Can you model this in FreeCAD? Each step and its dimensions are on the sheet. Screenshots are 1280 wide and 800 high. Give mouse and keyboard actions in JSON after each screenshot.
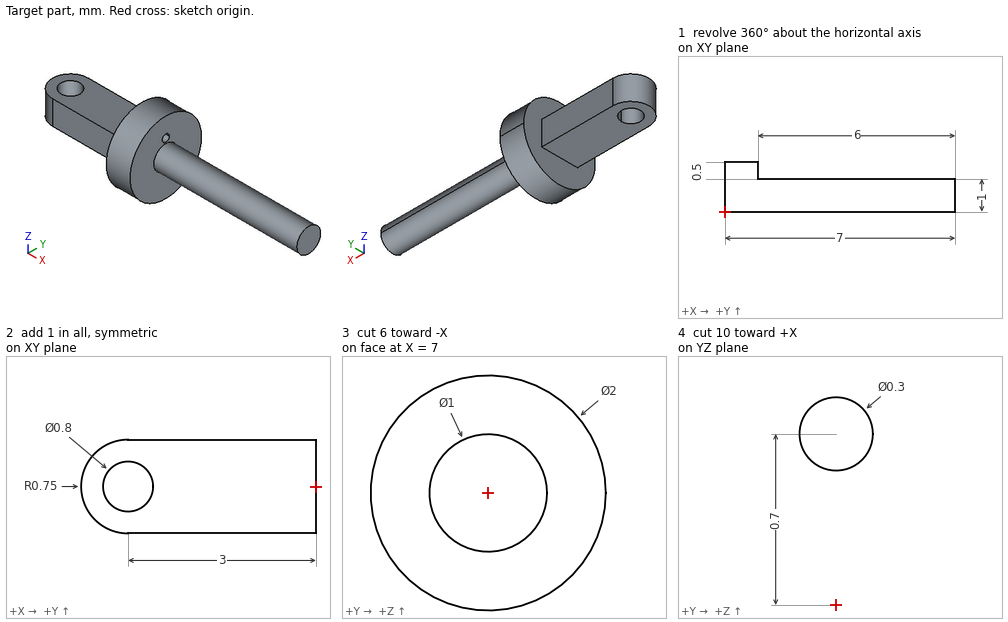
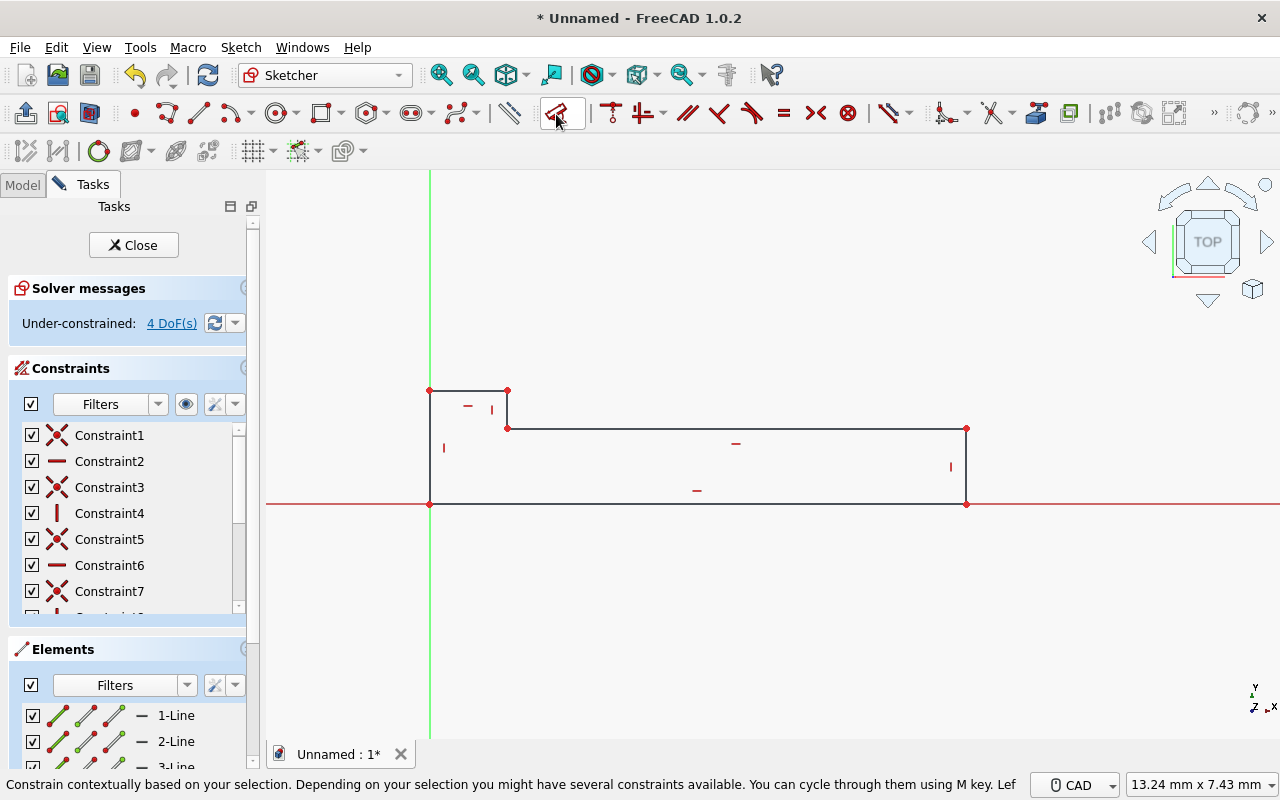
{"action": "left_click", "coordinate": [591, 504]}
{"action": "left_click", "coordinate": [698, 538]}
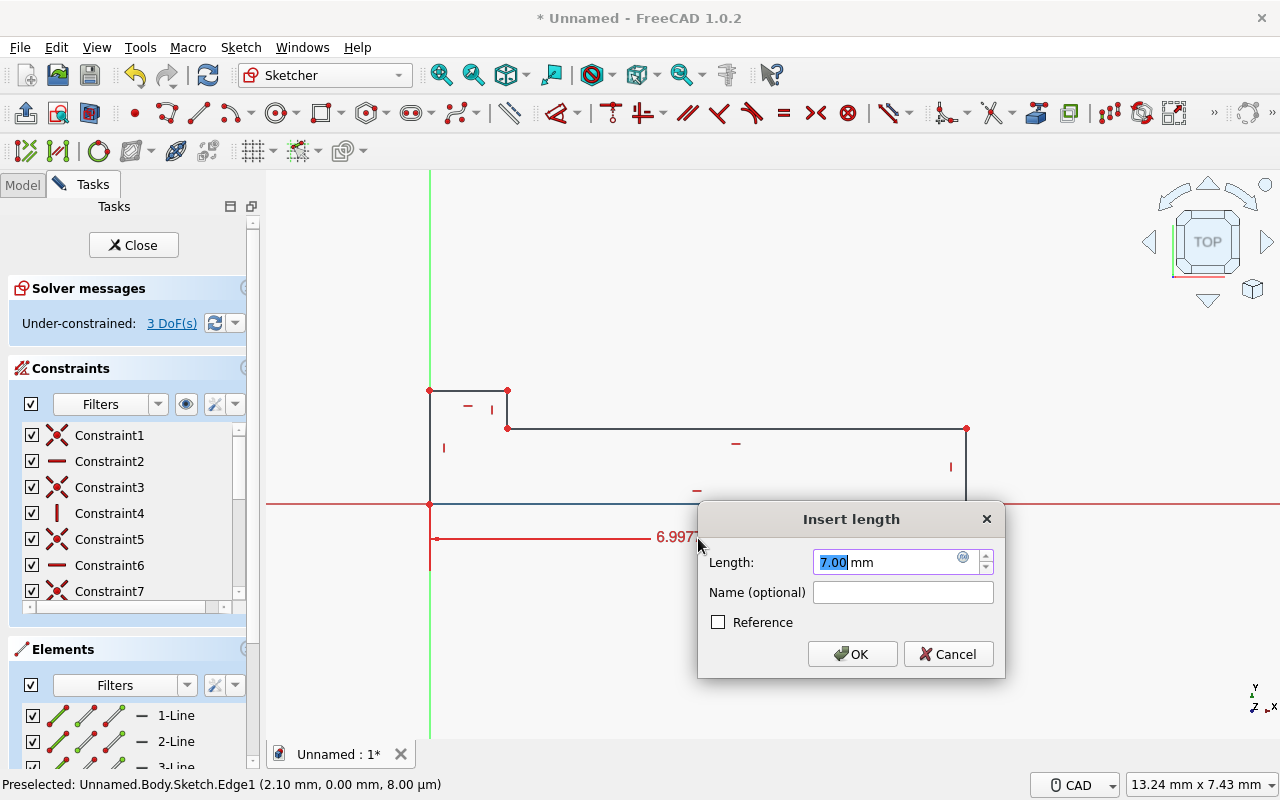
{"action": "type", "text": "7"}
{"action": "key", "text": "Return"}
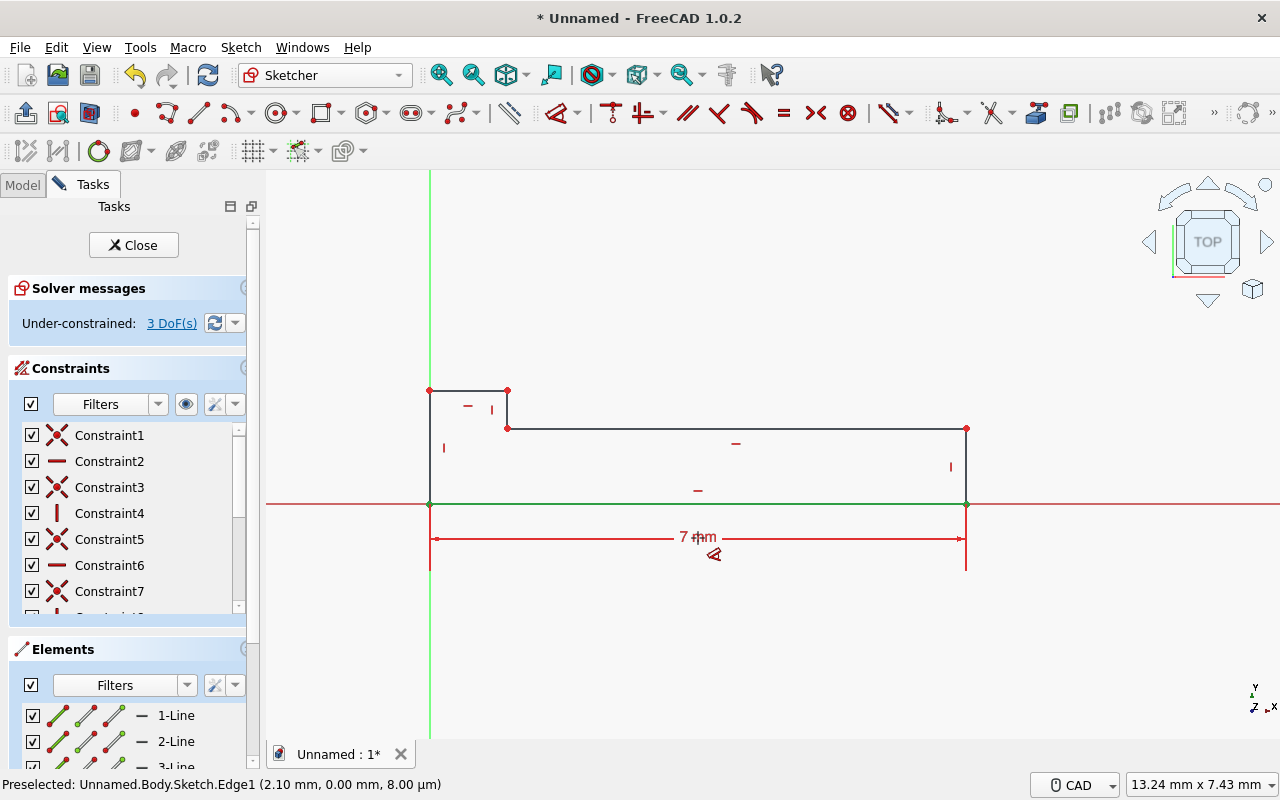
{"action": "left_click", "coordinate": [966, 482]}
{"action": "left_click", "coordinate": [1000, 467]}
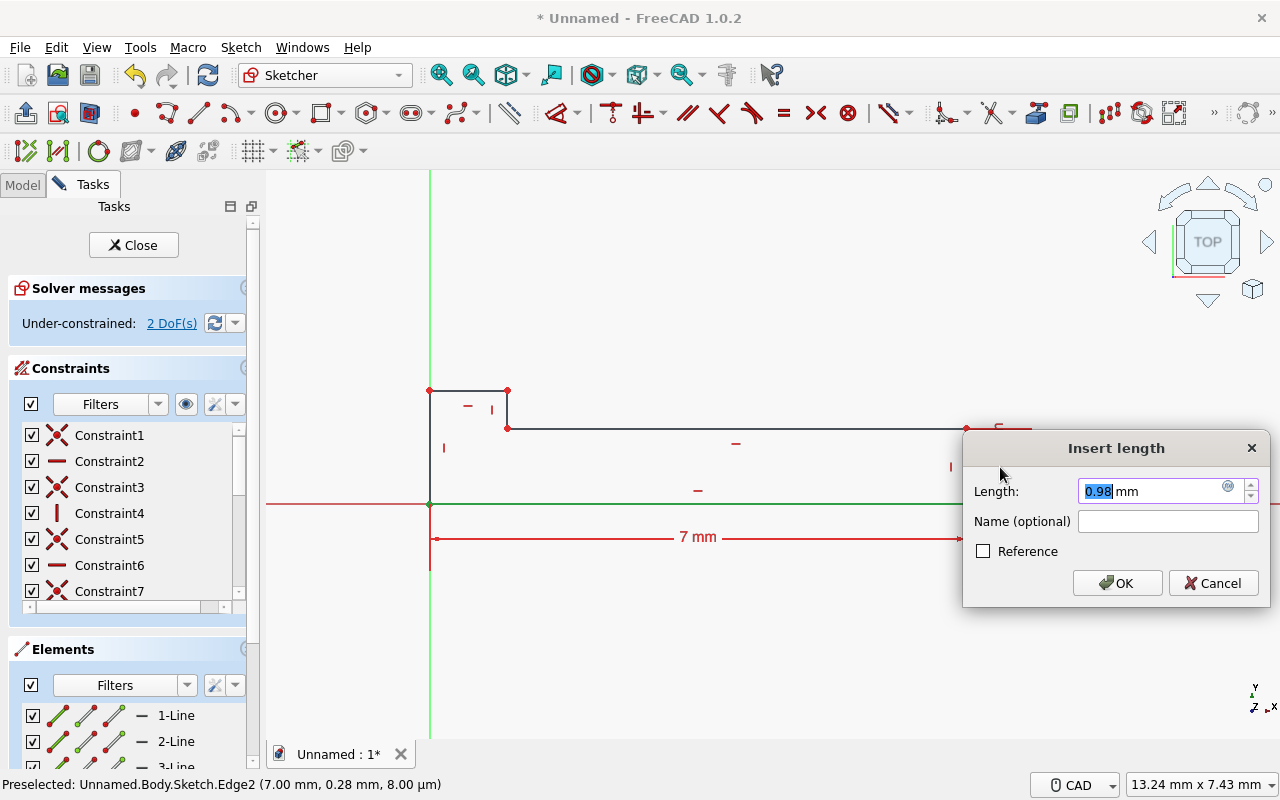
{"action": "type", "text": "1"}
{"action": "key", "text": "Return"}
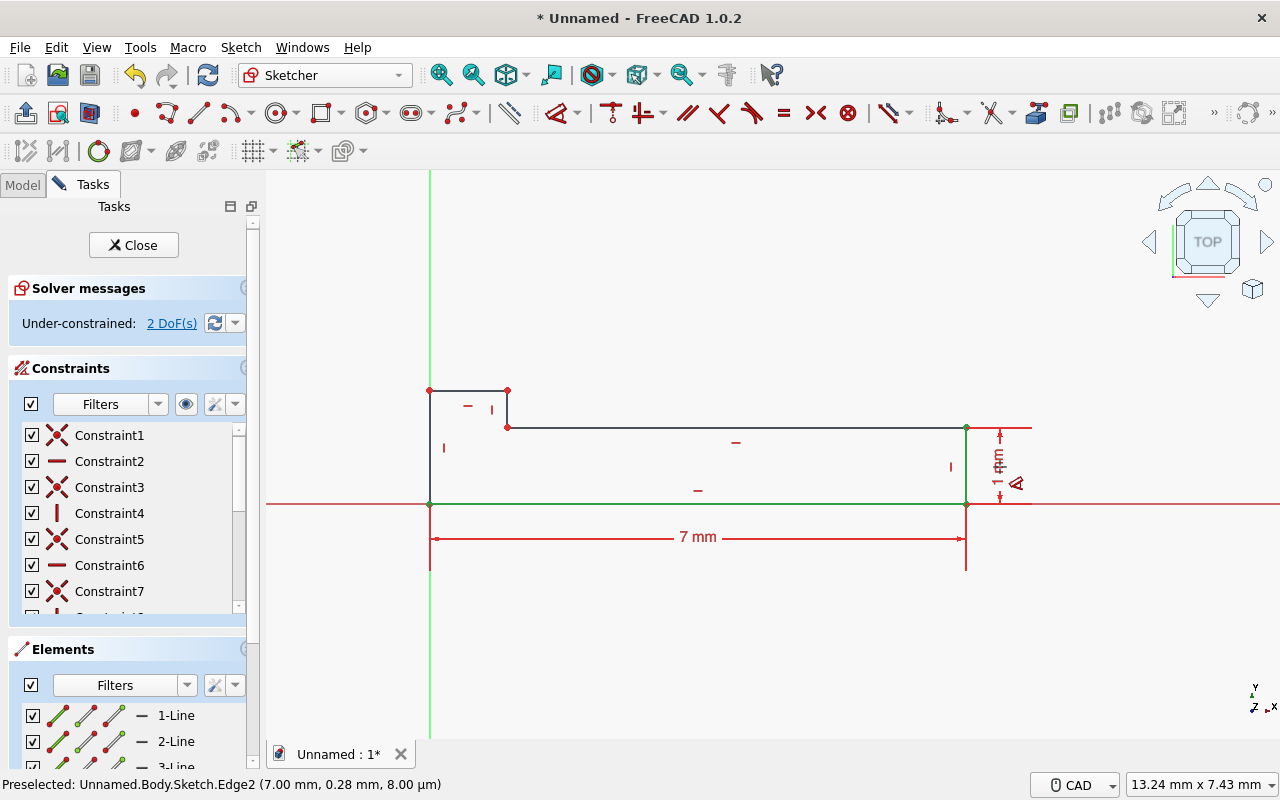
{"action": "left_click", "coordinate": [828, 428]}
{"action": "left_click", "coordinate": [737, 394]}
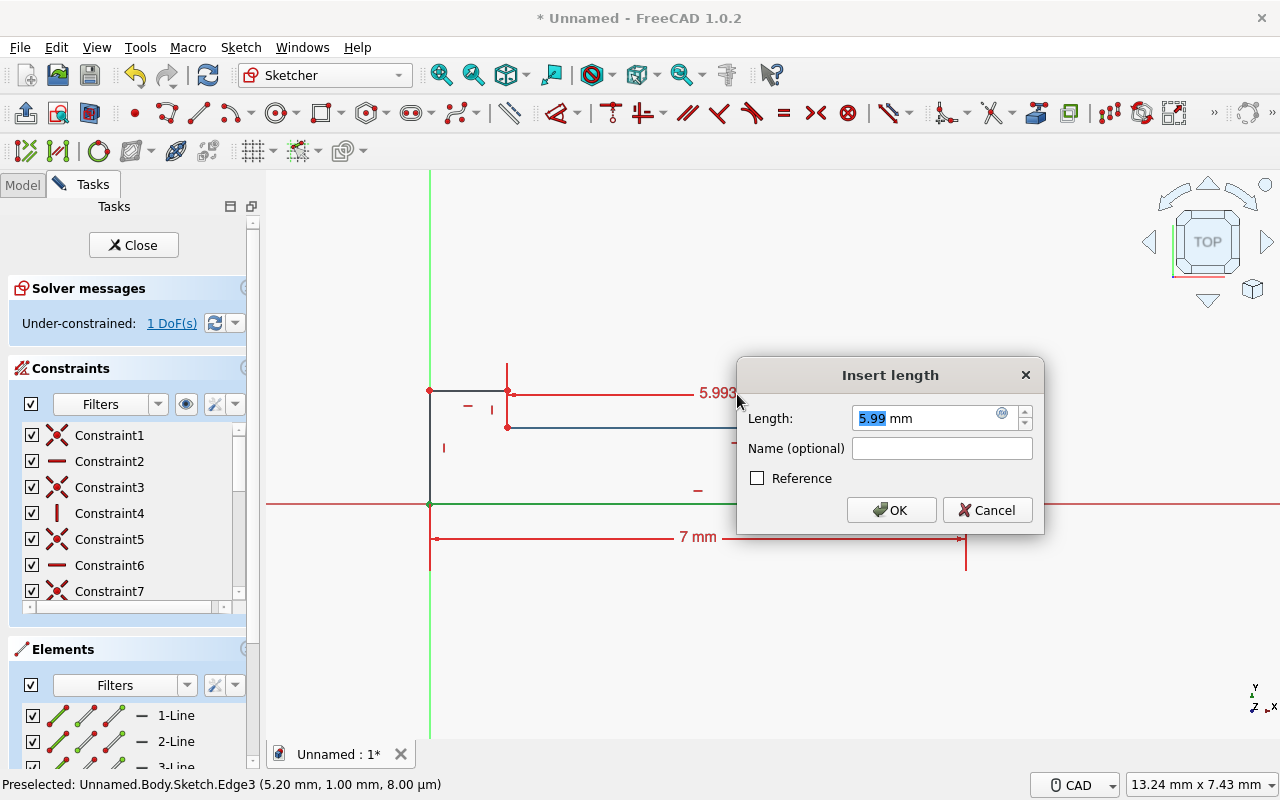
{"action": "type", "text": "6"}
{"action": "key", "text": "Return"}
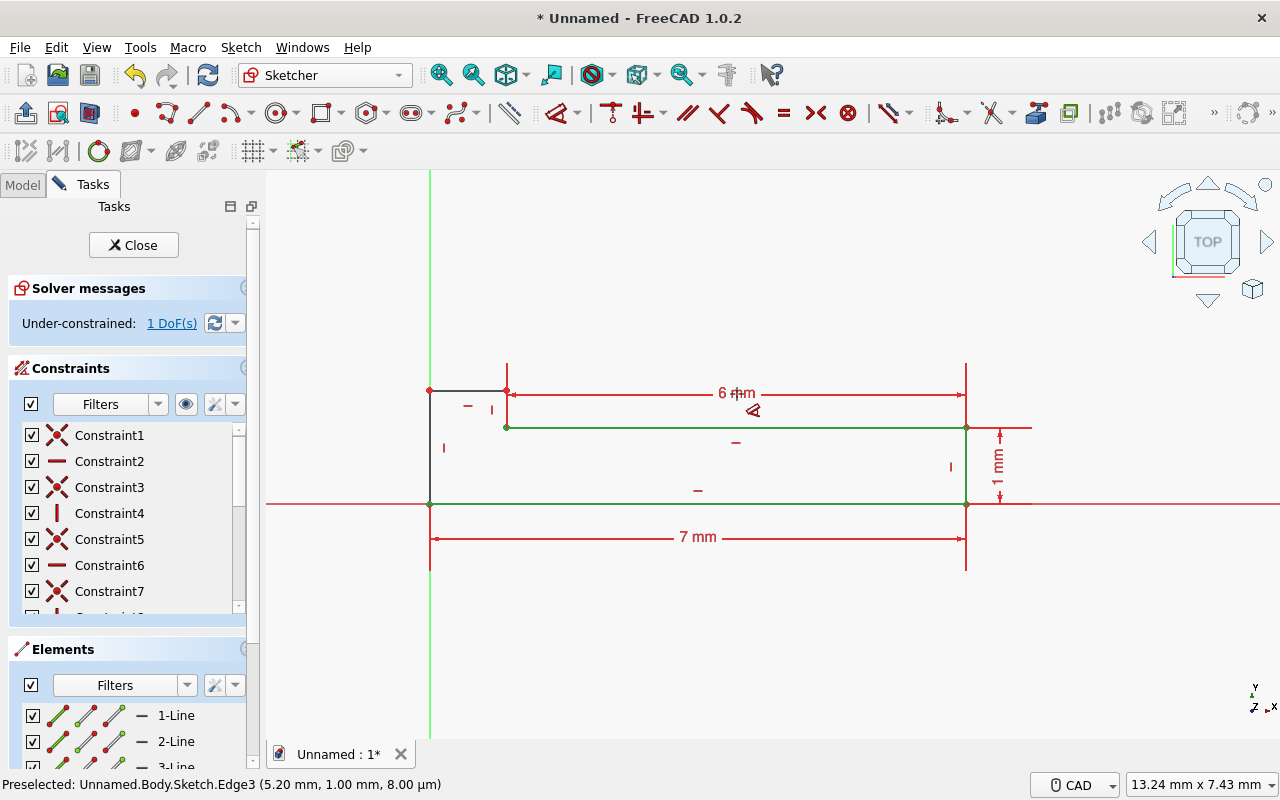
{"action": "scroll", "coordinate": [507, 417], "scroll_direction": "up", "scroll_amount": 2}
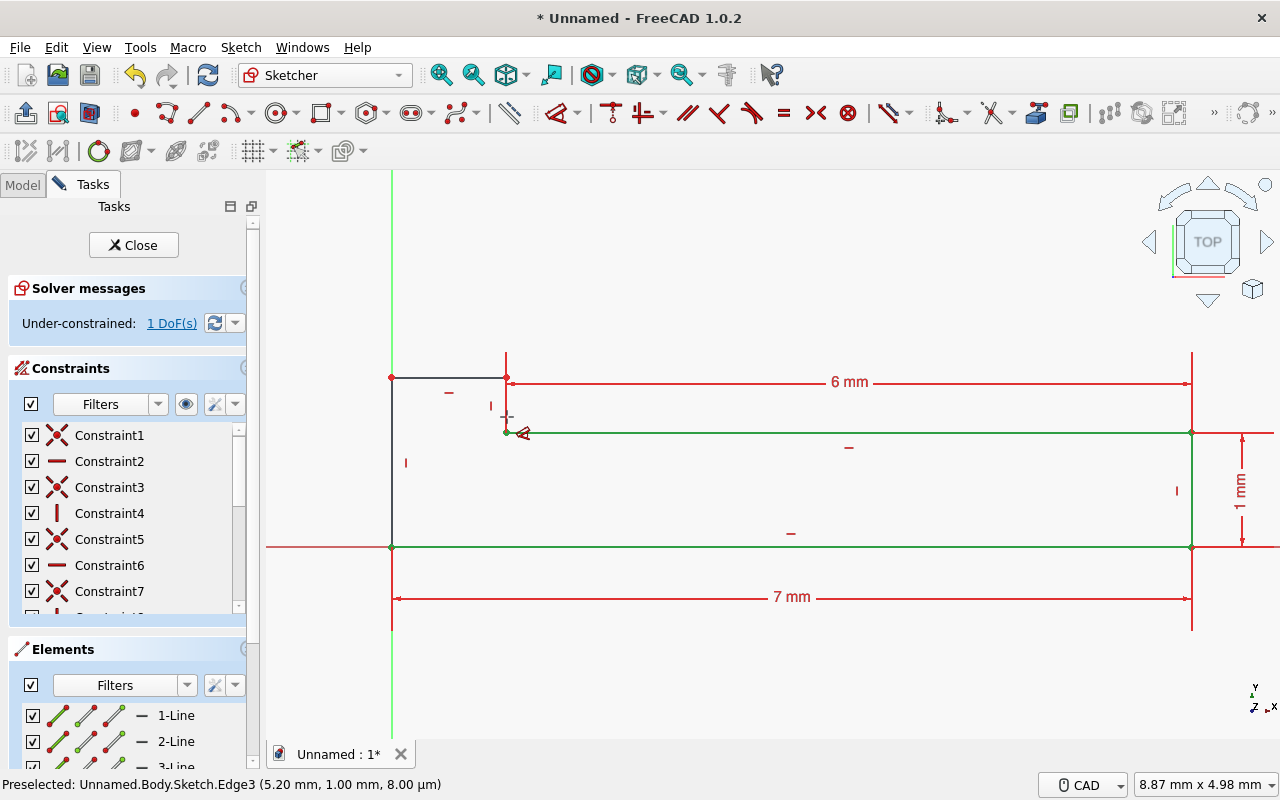
{"action": "left_click", "coordinate": [506, 416]}
{"action": "left_click", "coordinate": [472, 405]}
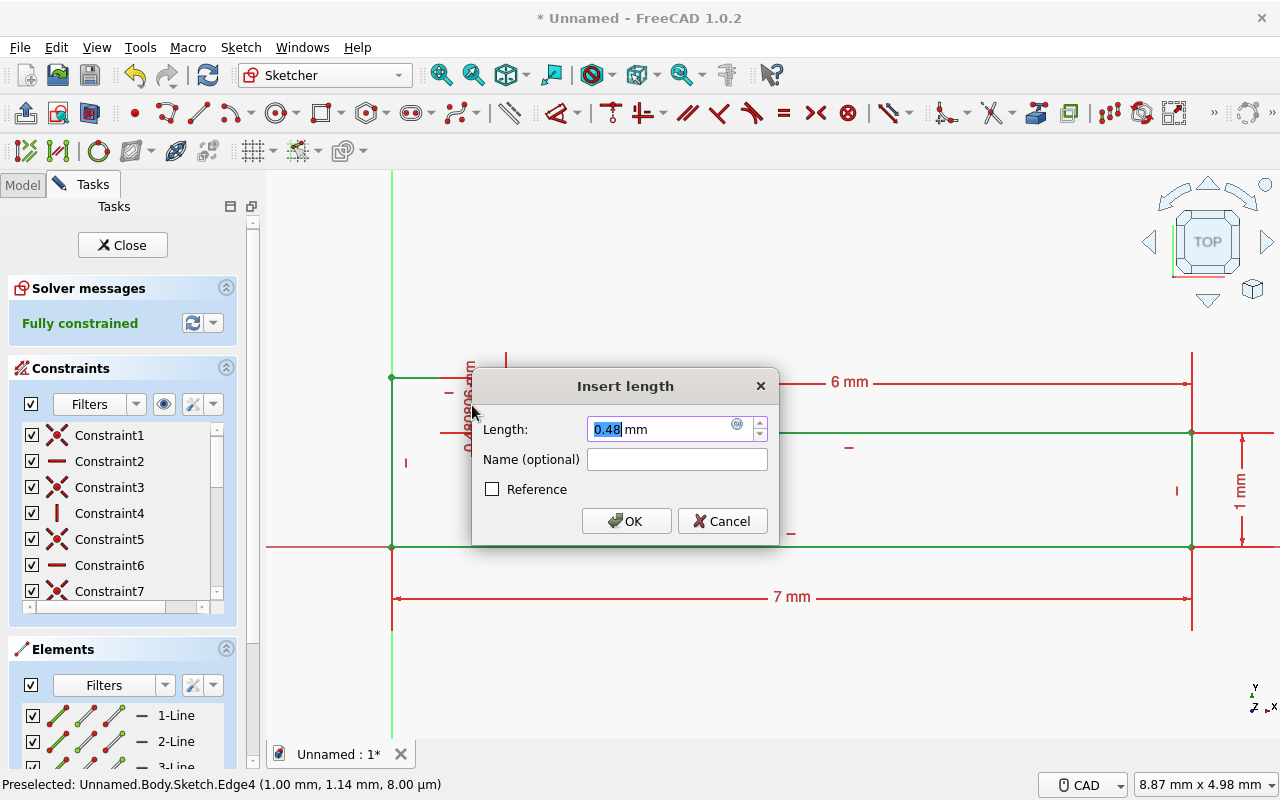
{"action": "type", "text": "0.5"}
{"action": "key", "text": "Return"}
{"action": "key", "text": "Escape"}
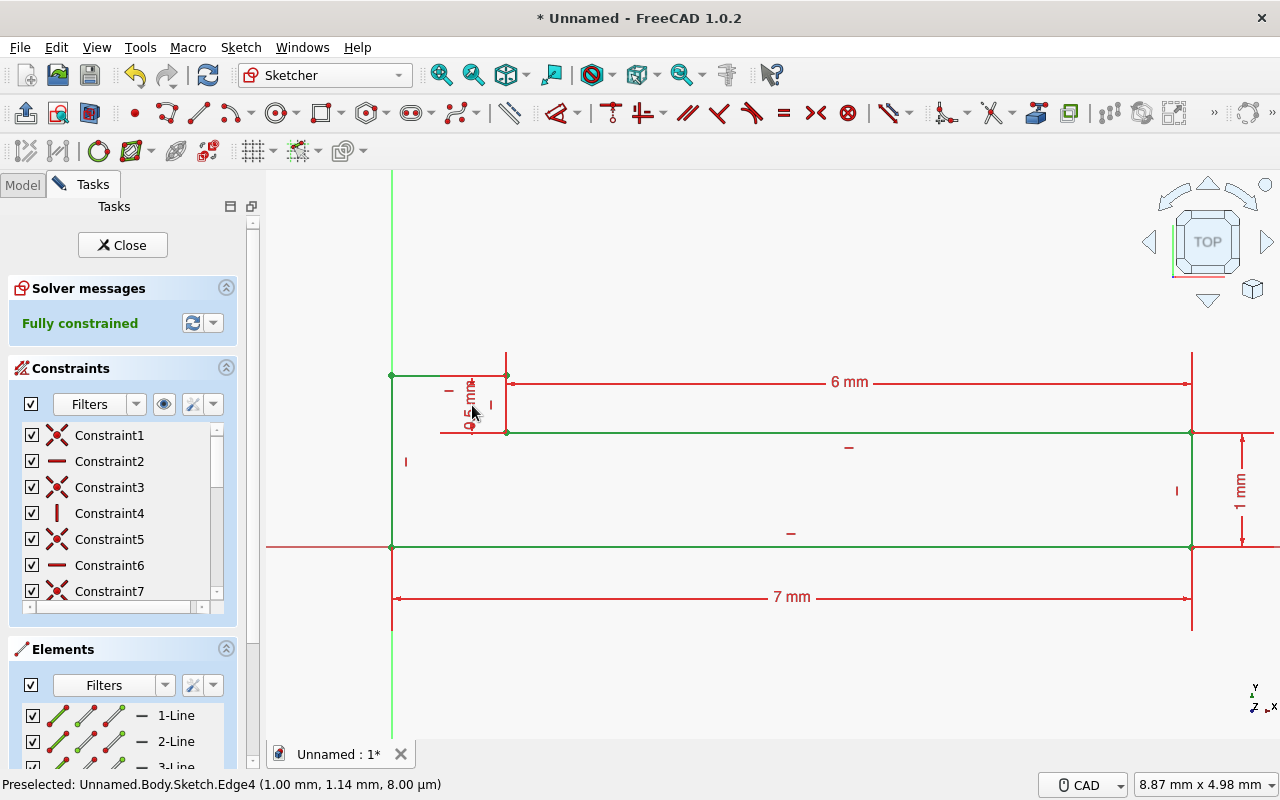
{"action": "left_click", "coordinate": [123, 245]}